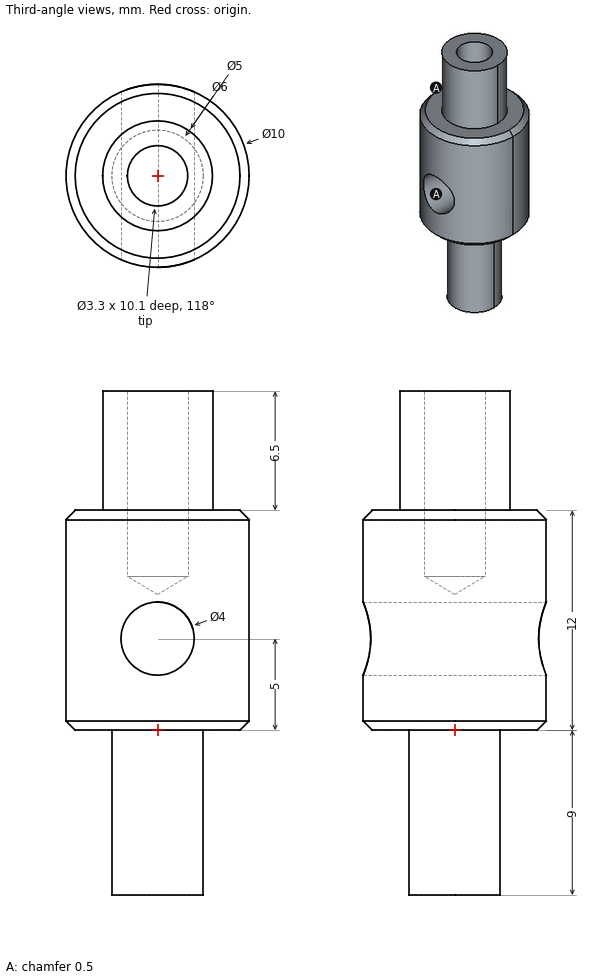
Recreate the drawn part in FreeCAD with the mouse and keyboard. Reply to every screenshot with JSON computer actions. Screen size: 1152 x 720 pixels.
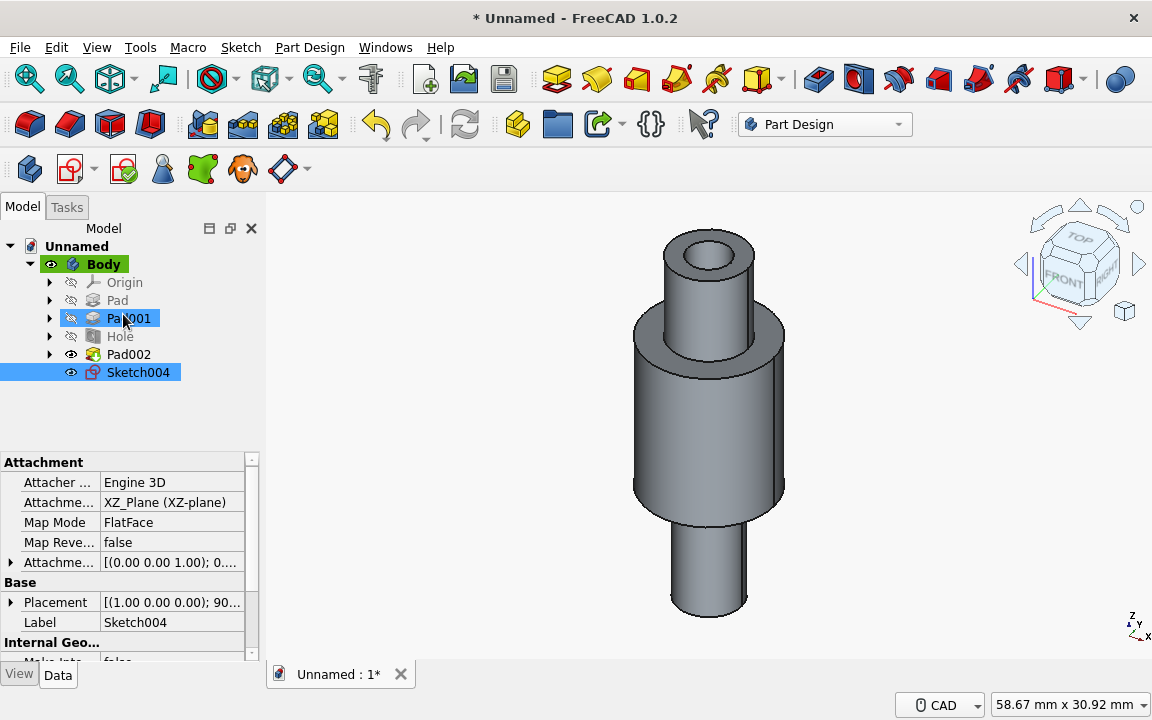
{"action": "left_click", "coordinate": [820, 80]}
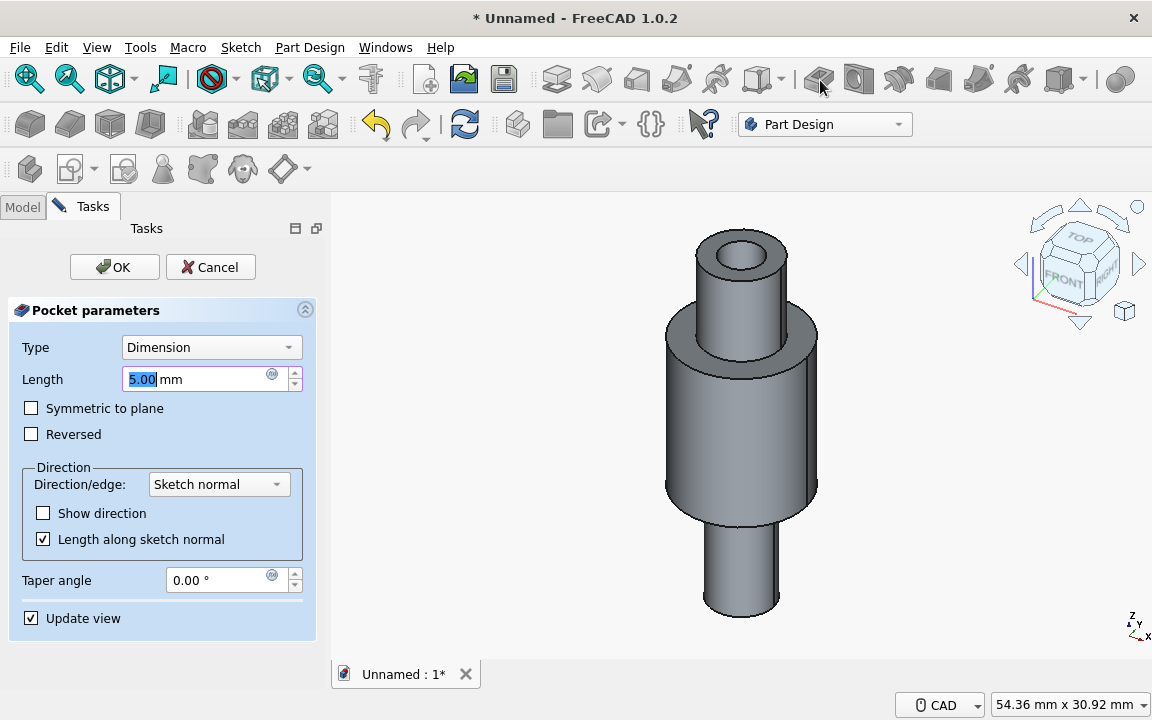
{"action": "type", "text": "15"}
{"action": "key", "text": "Tab"}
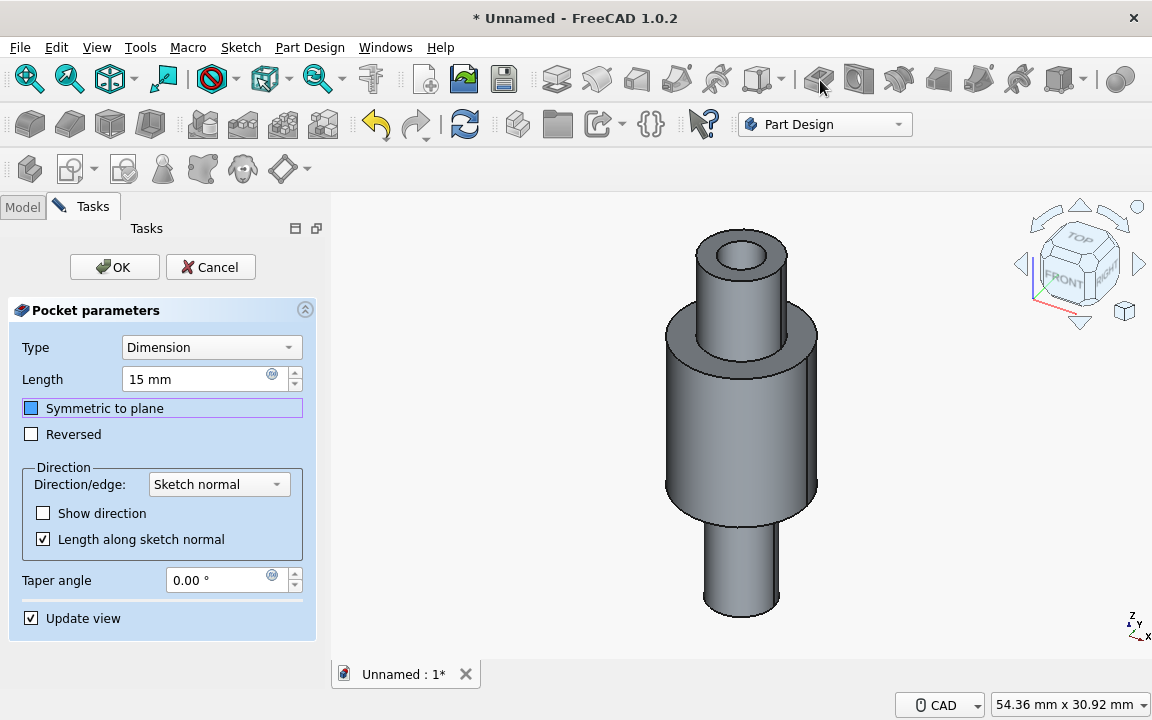
{"action": "left_click", "coordinate": [30, 408]}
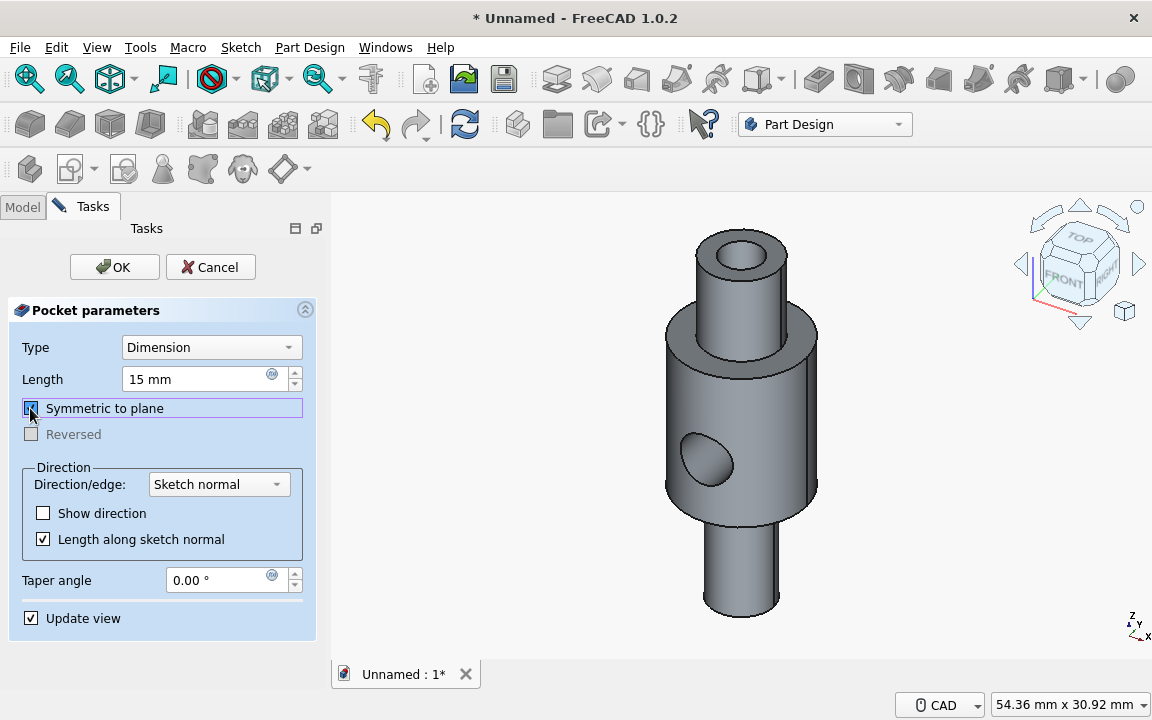
{"action": "left_click", "coordinate": [115, 267]}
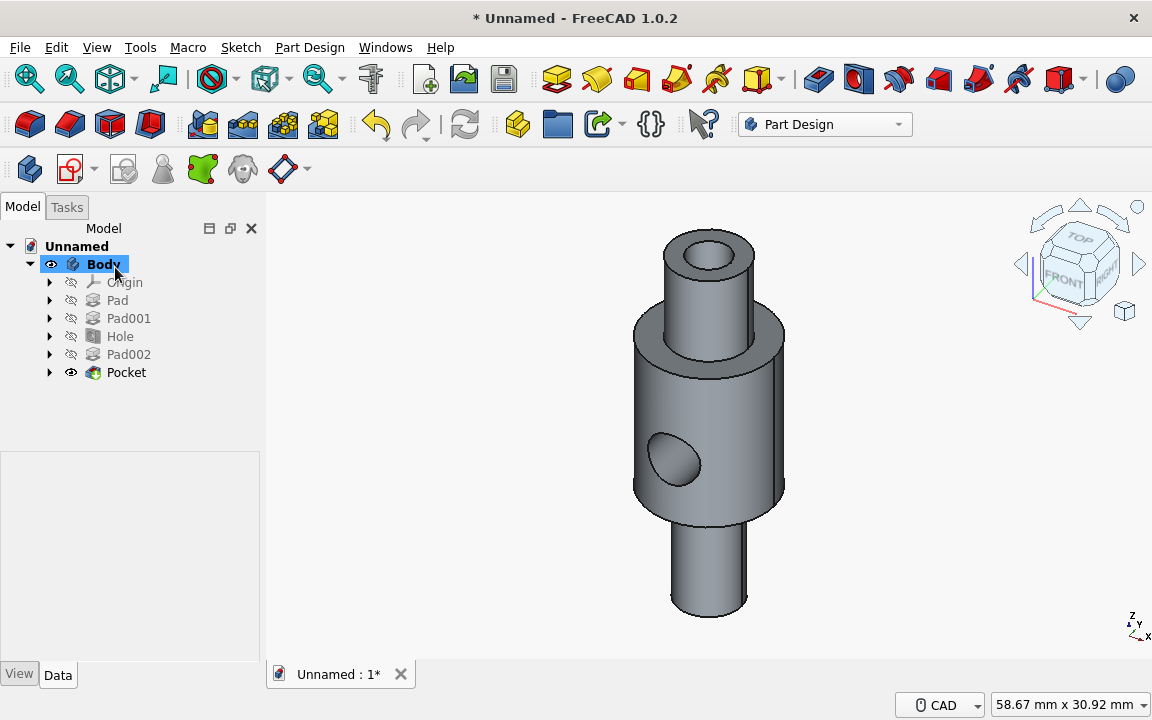
{"action": "left_click", "coordinate": [634, 339]}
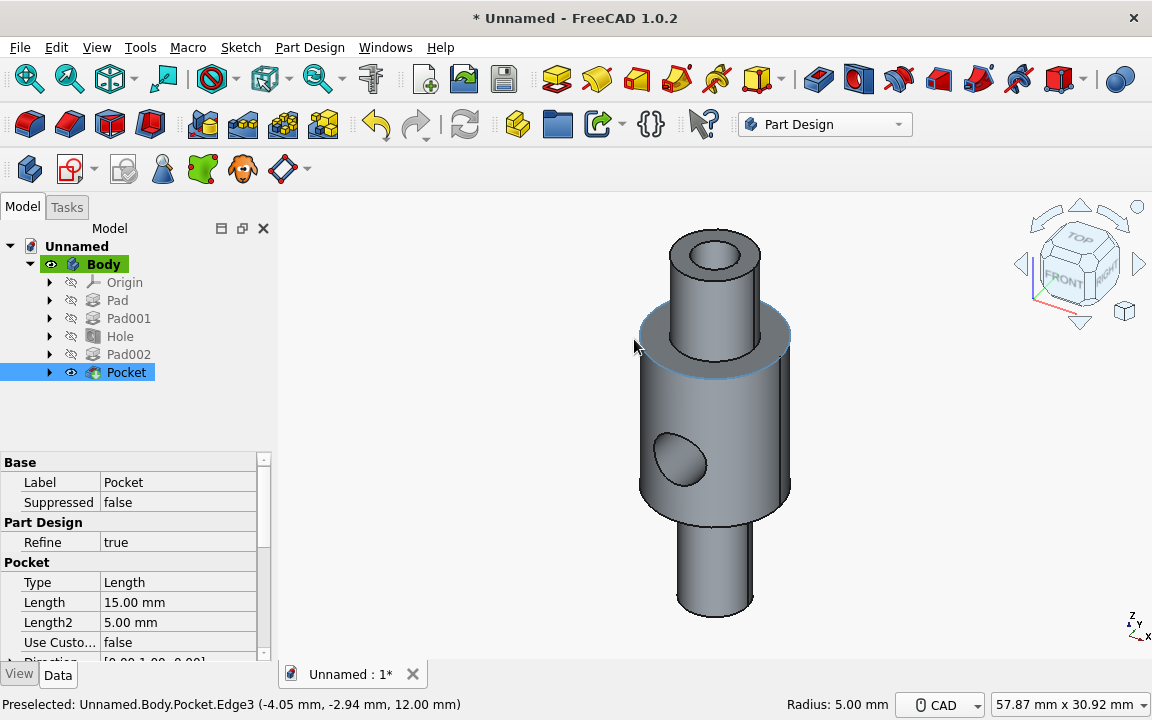
{"action": "key", "text": "0"}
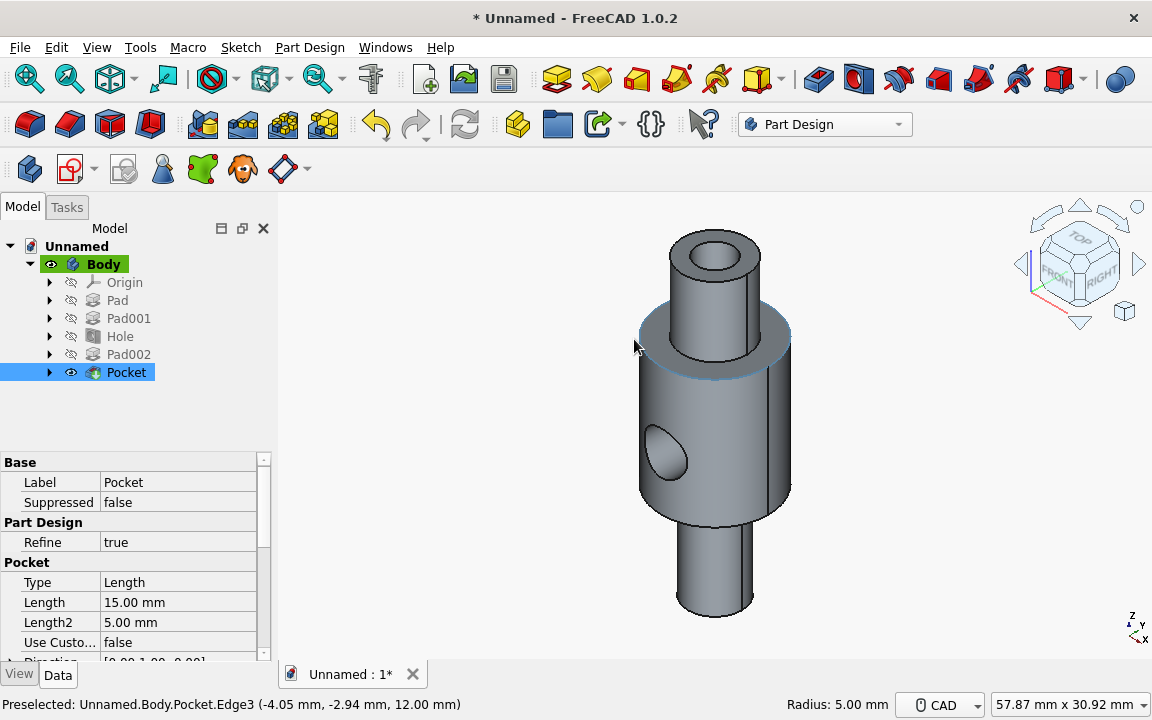
{"action": "key", "text": "2"}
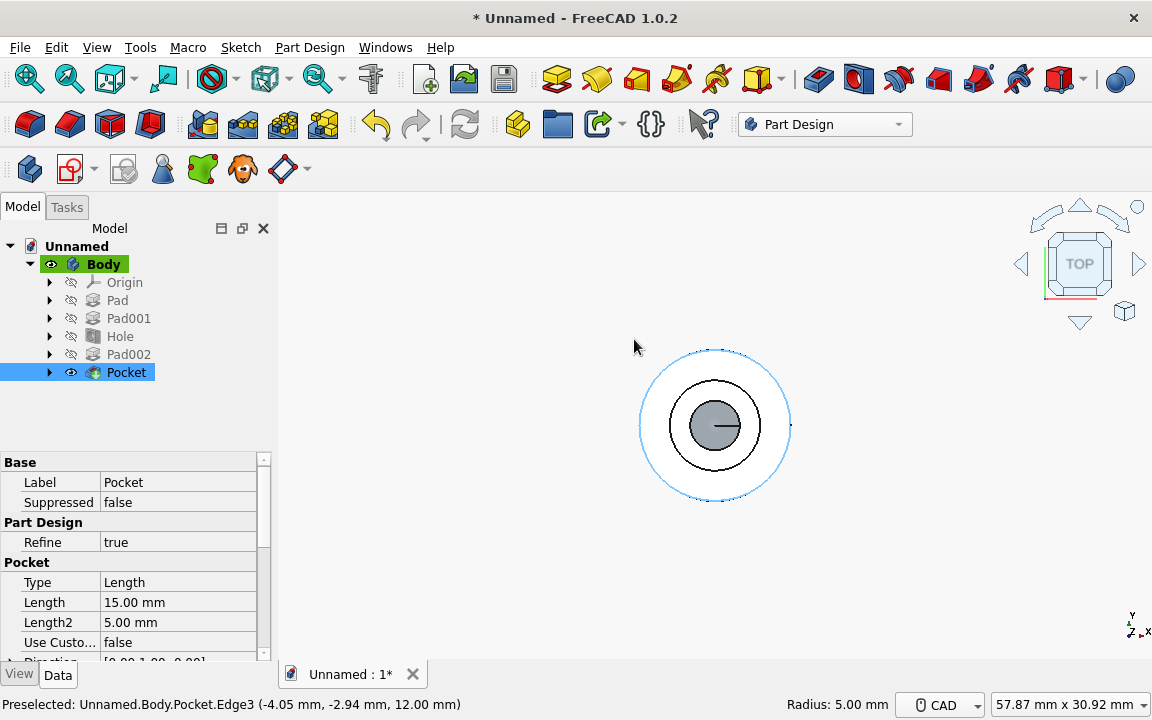
{"action": "left_click", "coordinate": [30, 80]}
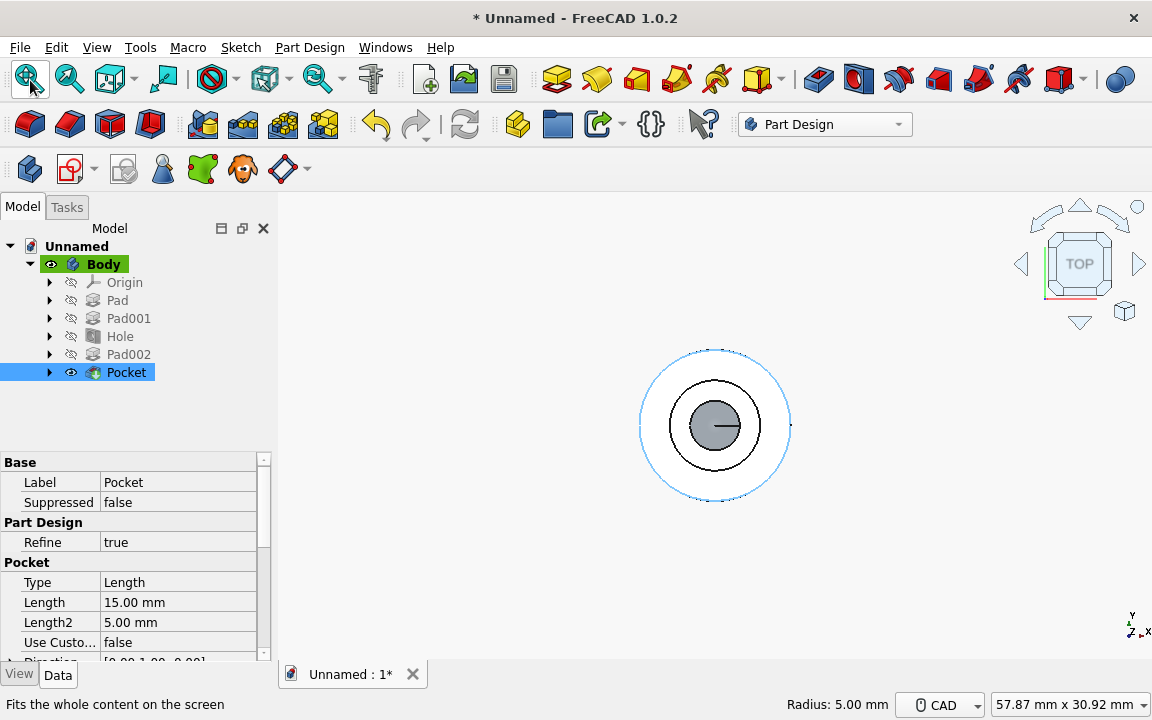
{"action": "key", "text": "1"}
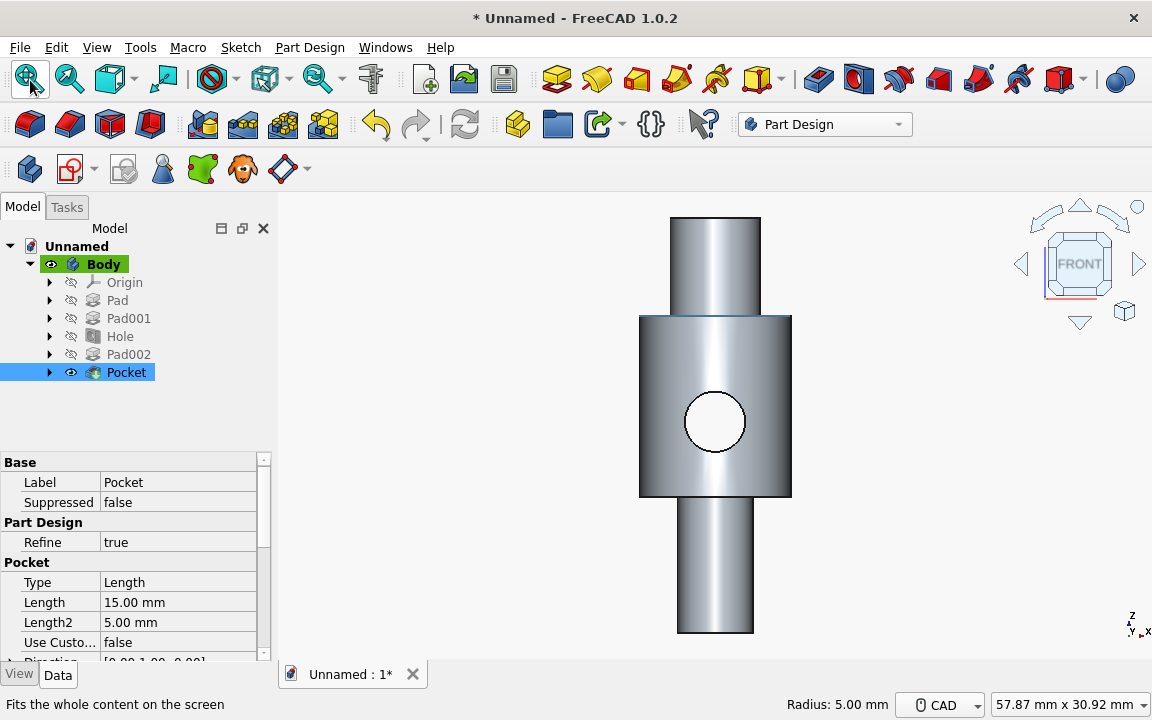
{"action": "left_click", "coordinate": [654, 496], "text": "ctrl"}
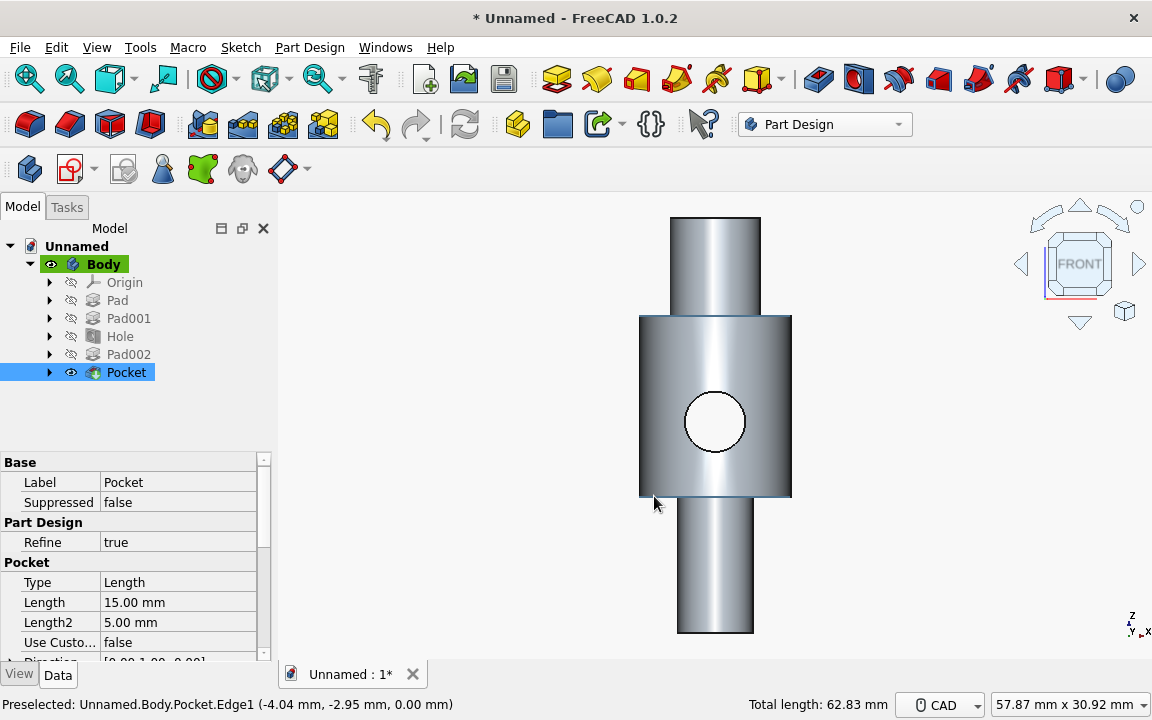
{"action": "left_click", "coordinate": [70, 124]}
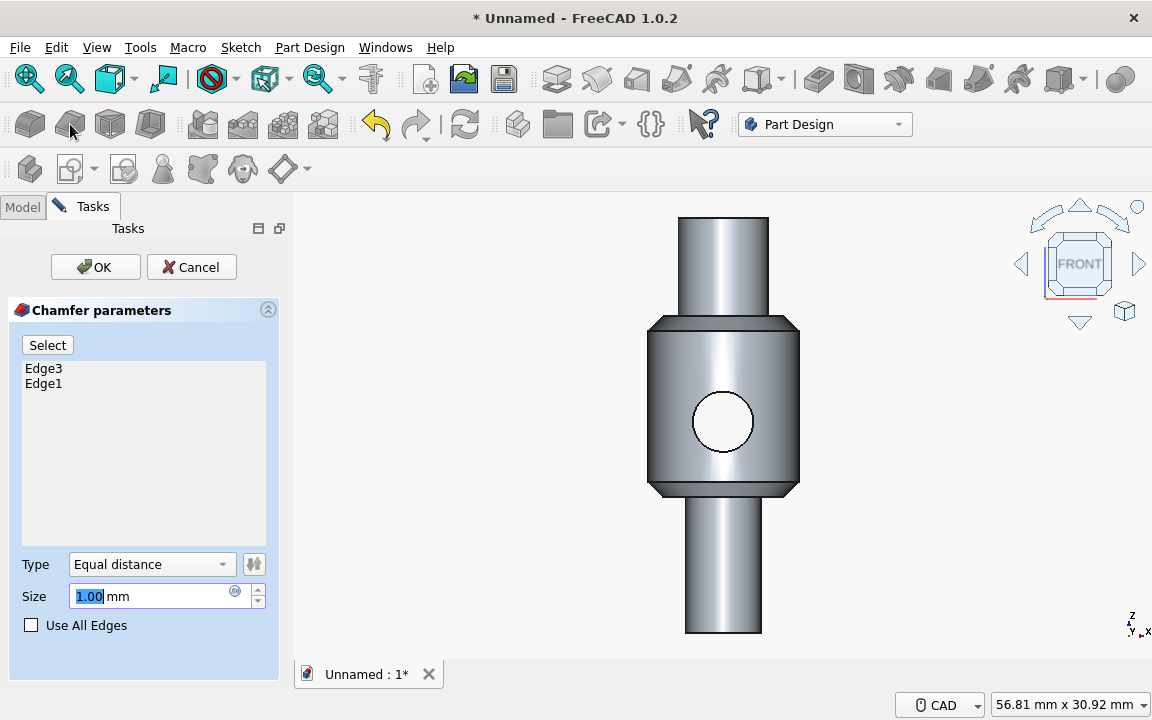
{"action": "type", "text": "0.5"}
{"action": "key", "text": "Tab"}